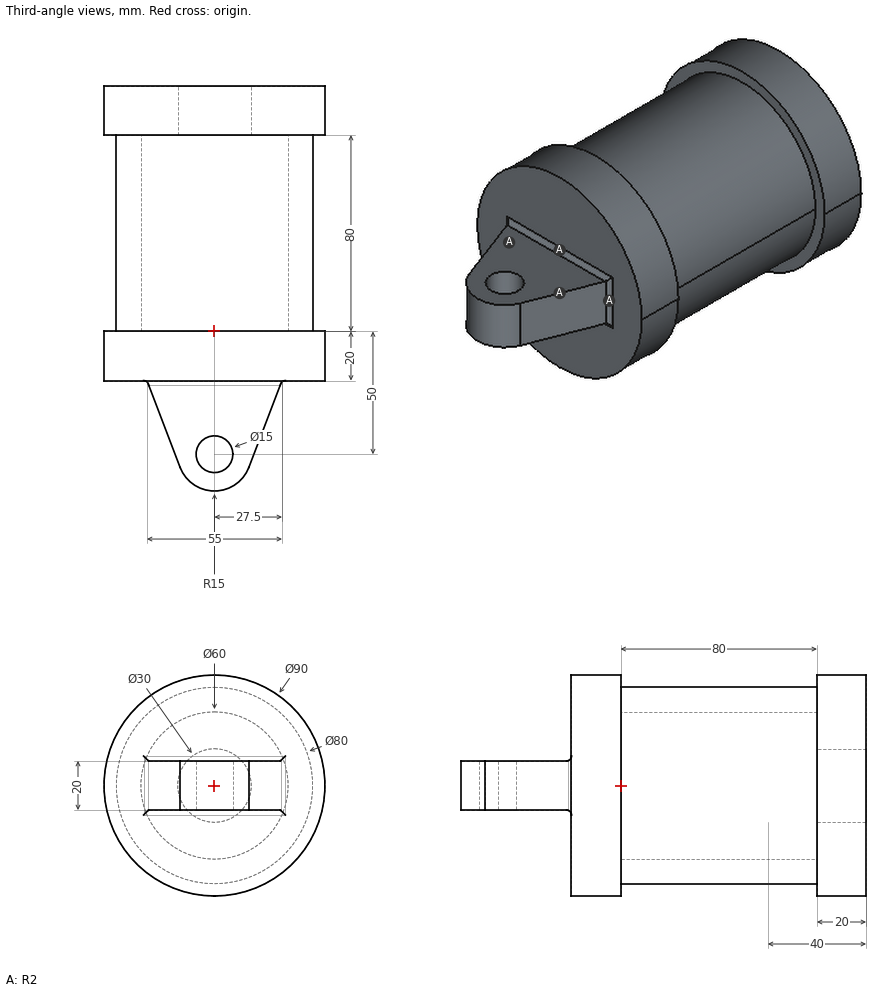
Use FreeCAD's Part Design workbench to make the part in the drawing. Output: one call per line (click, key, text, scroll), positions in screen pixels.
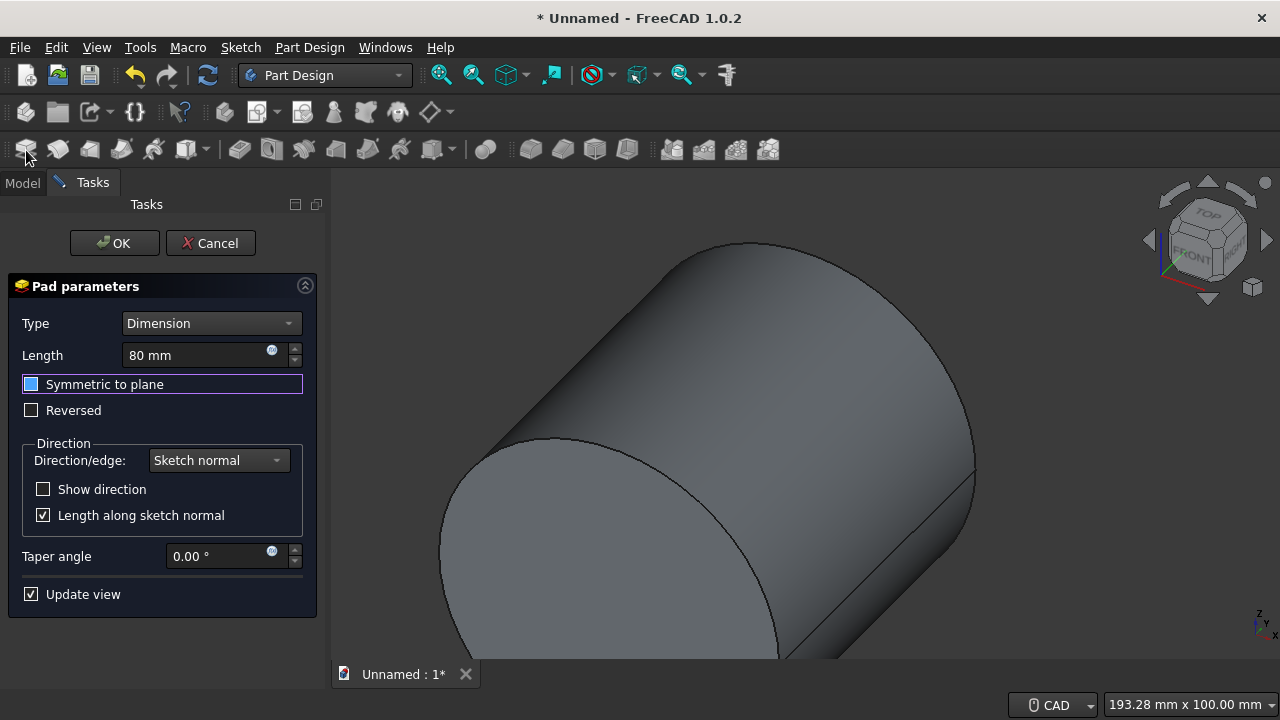
click(30, 410)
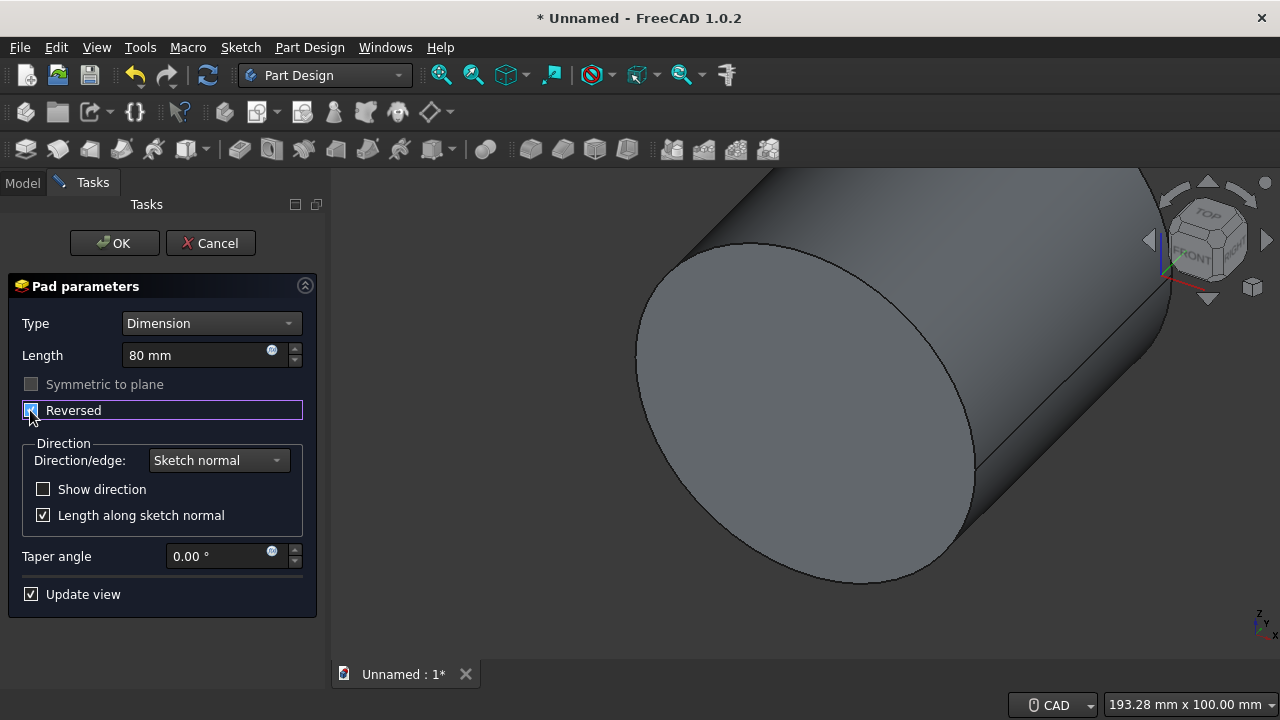
click(115, 243)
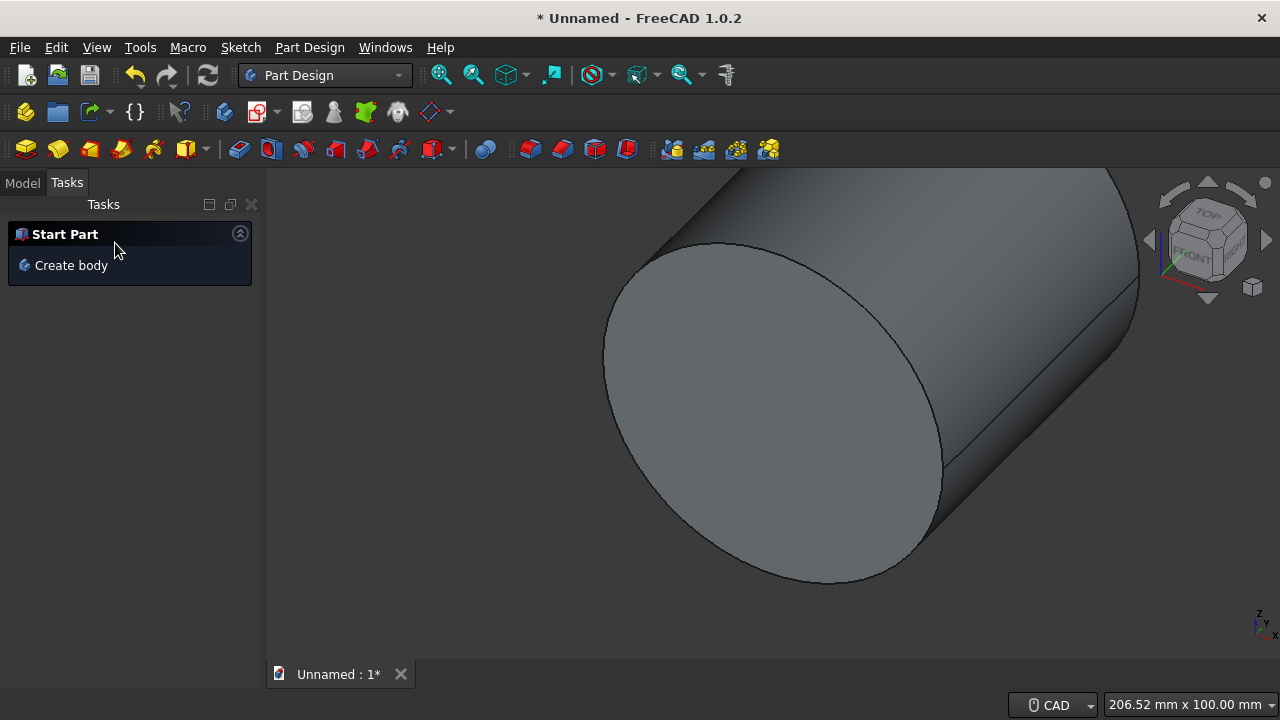
key(v)
key(f)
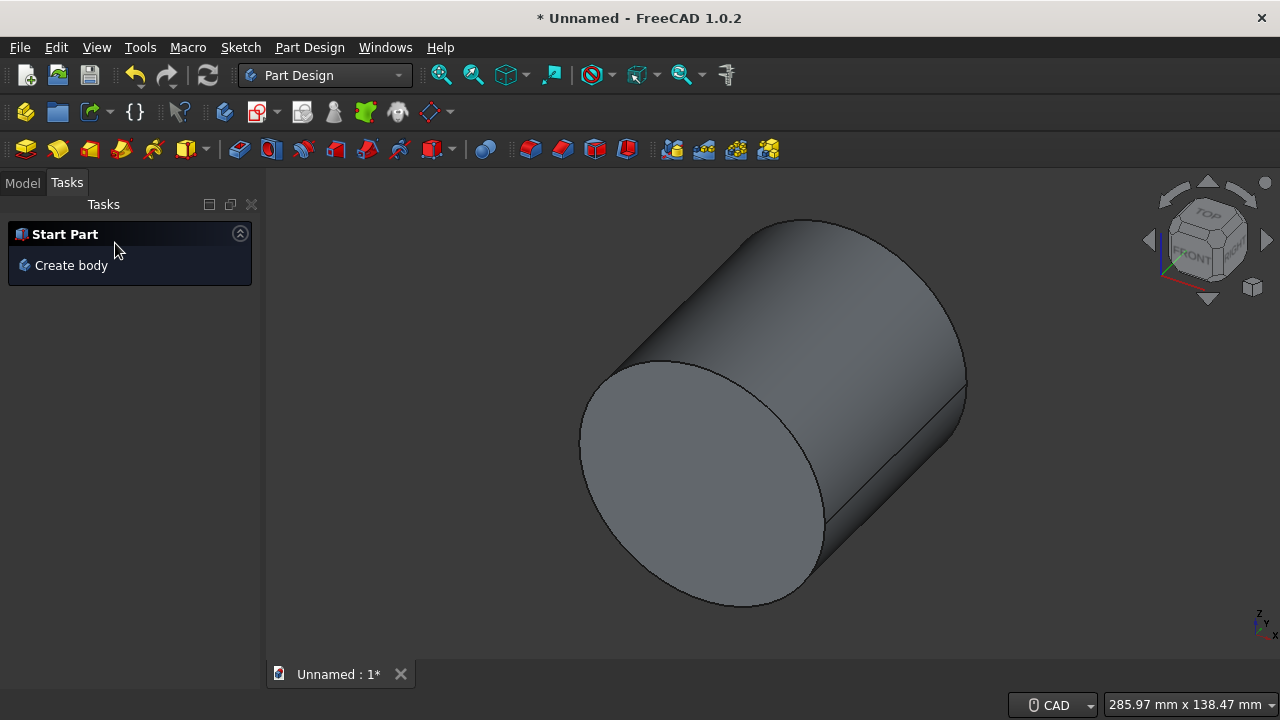
click(258, 112)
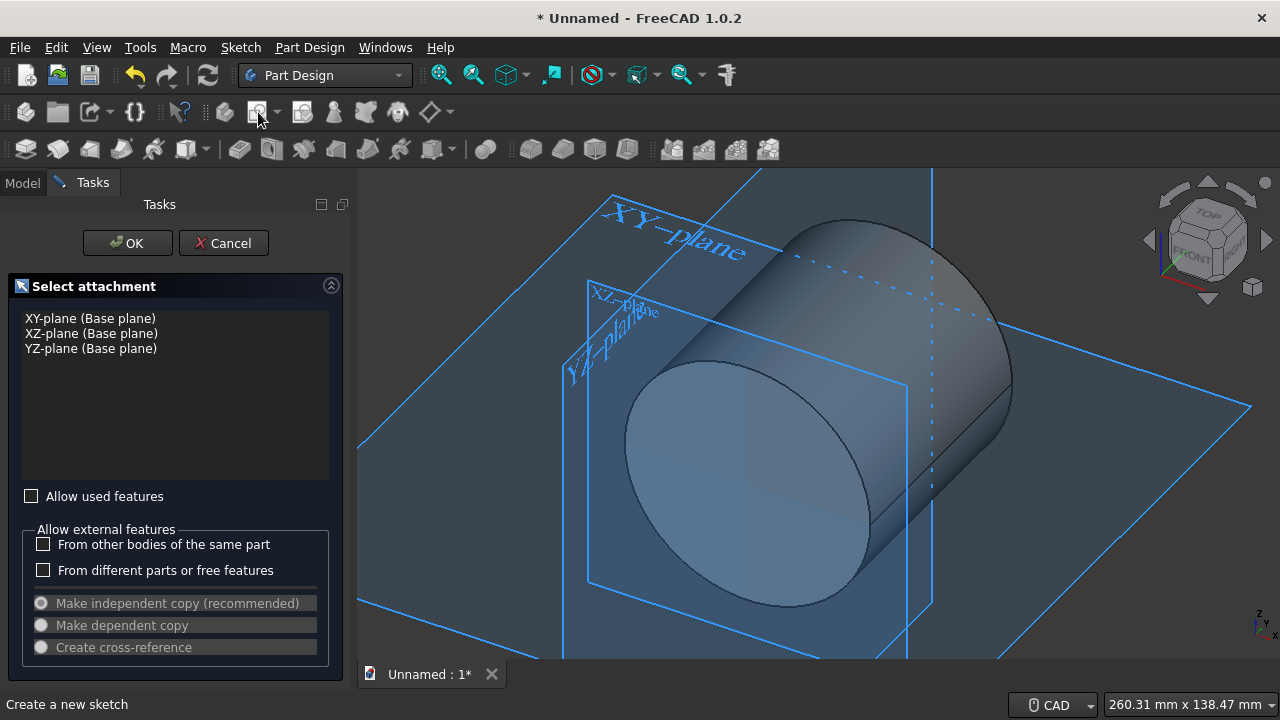
click(82, 334)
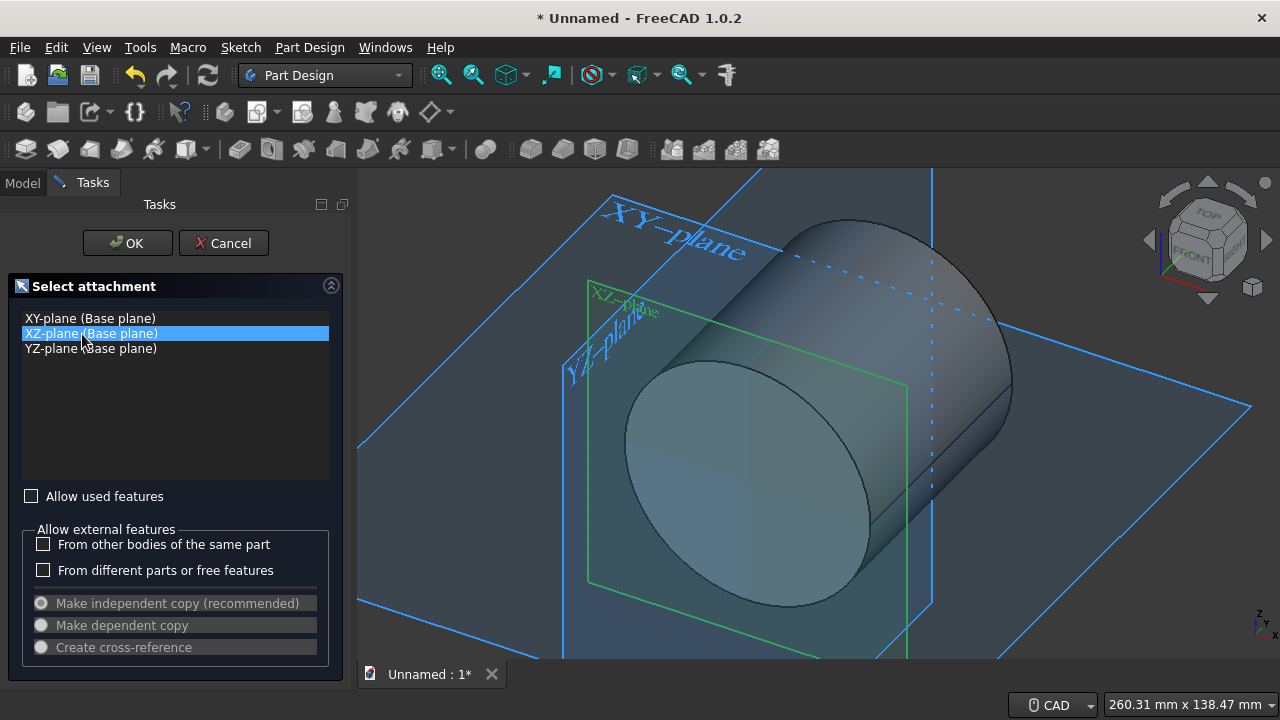
click(128, 243)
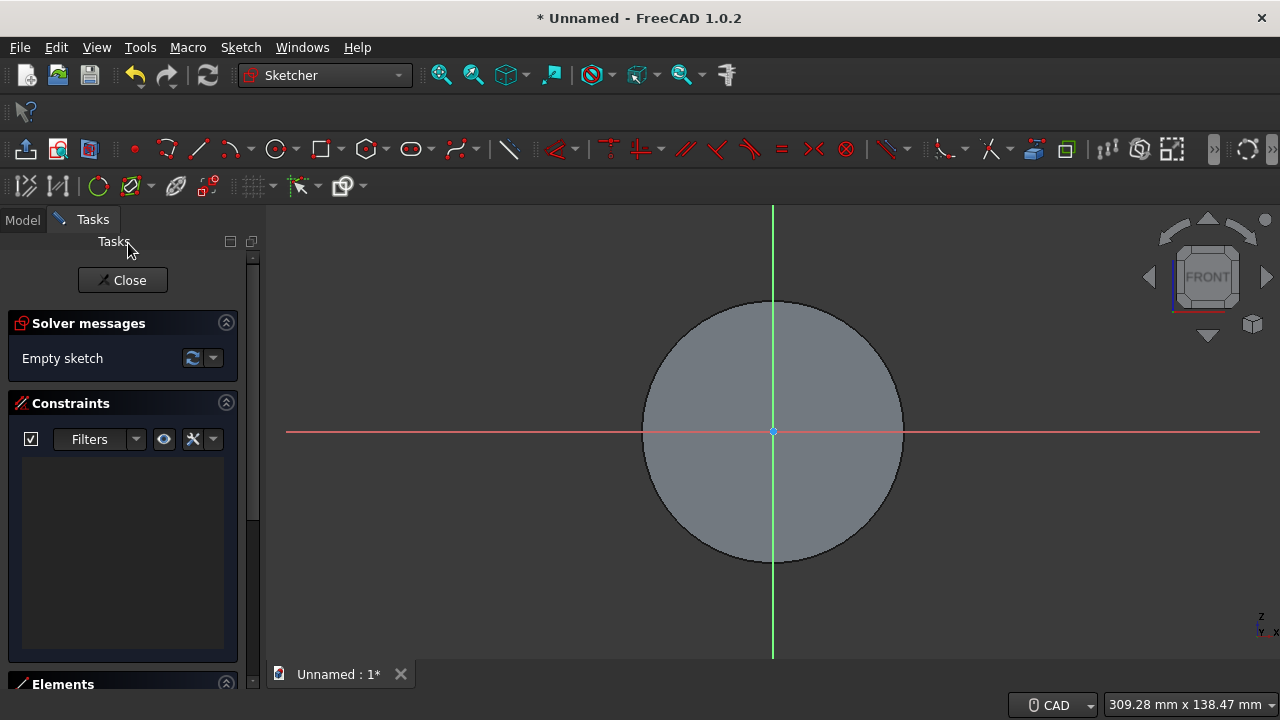
key(g)
key(c)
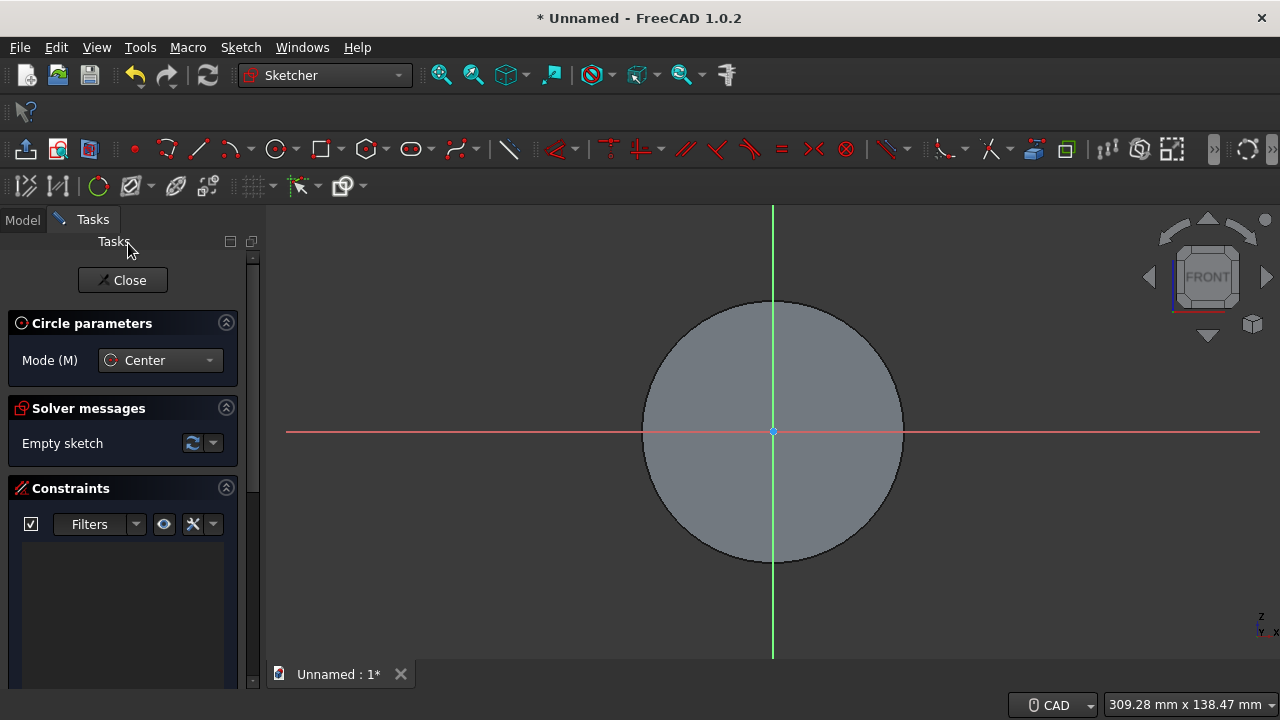
click(773, 432)
move(877, 328)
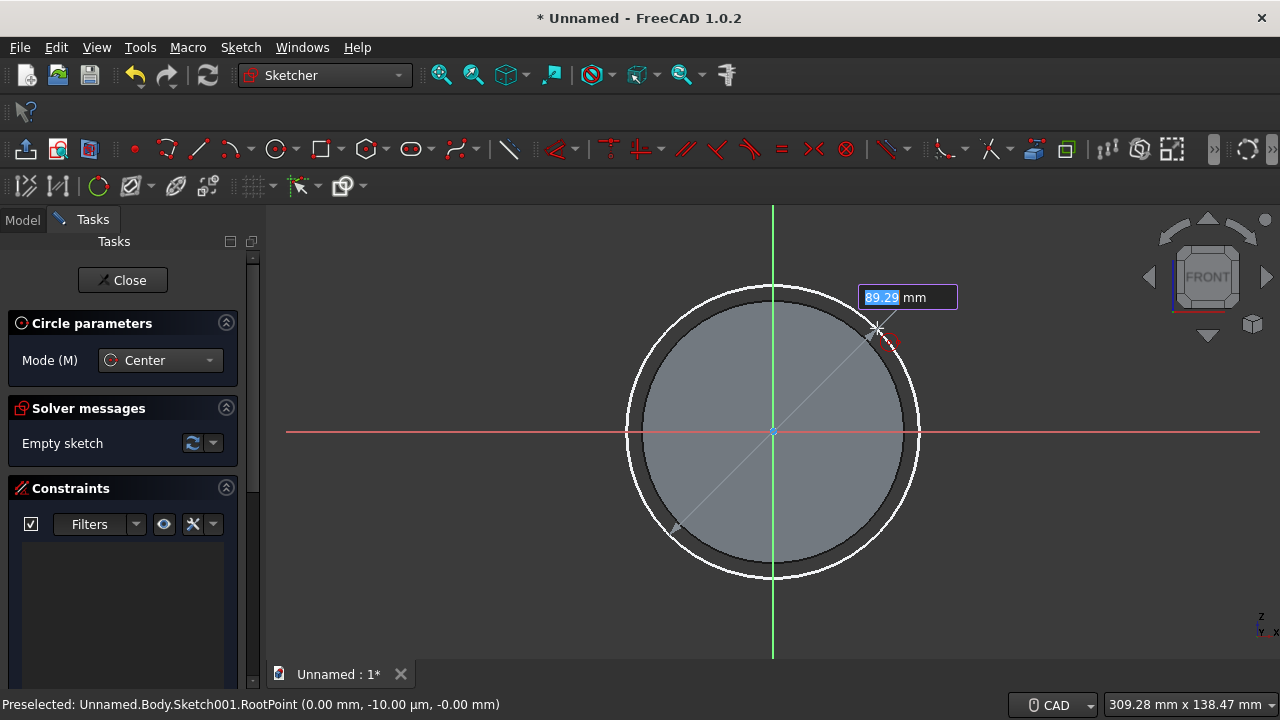
text(90)
key(Return)
key(Escape)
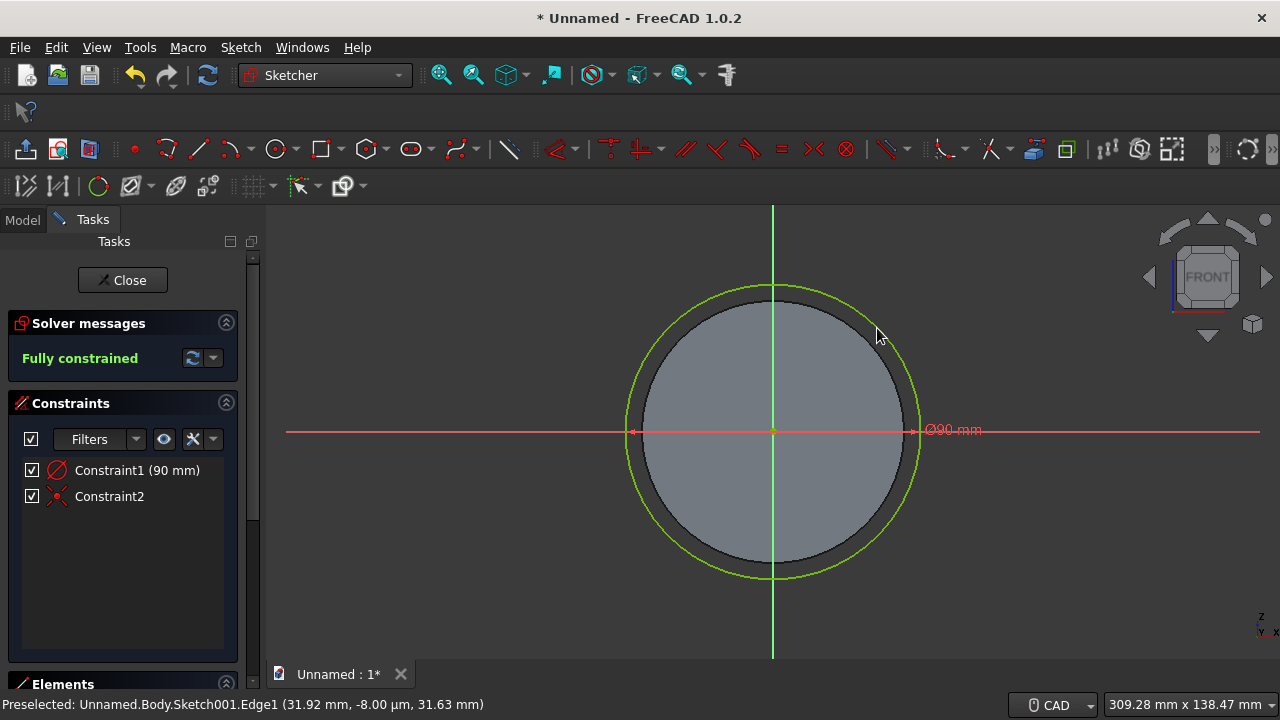
click(123, 280)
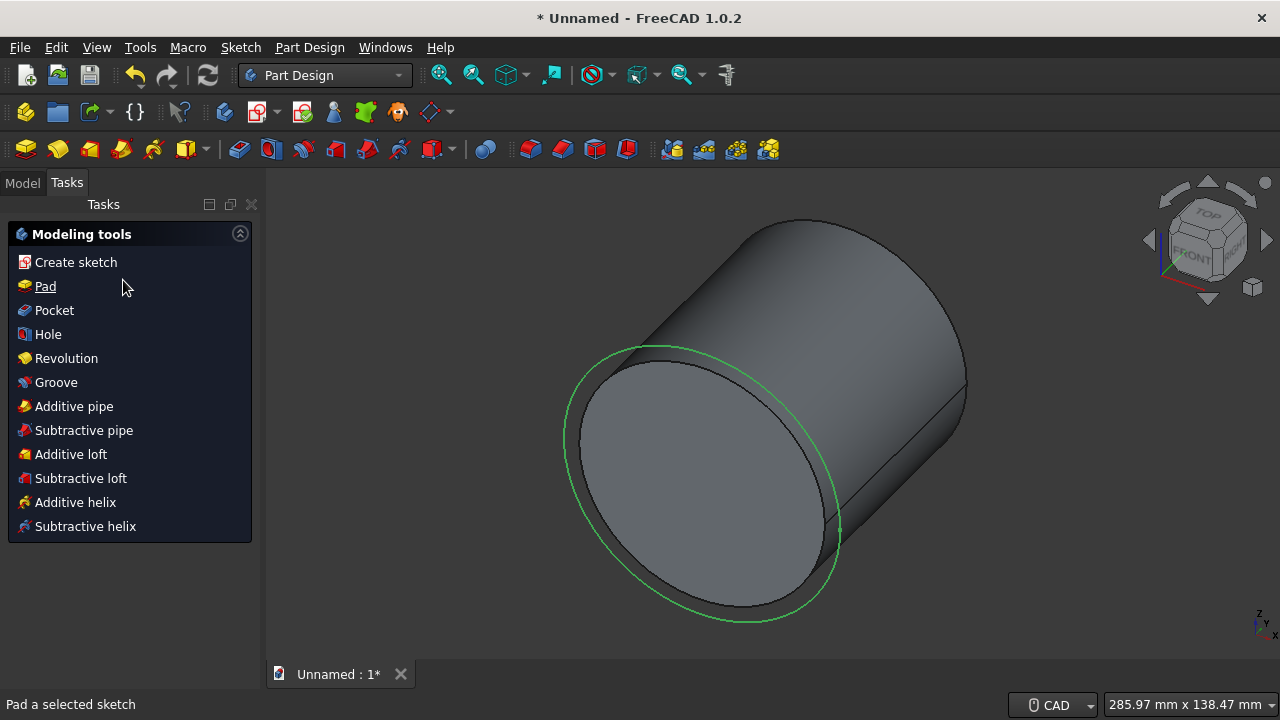
click(26, 150)